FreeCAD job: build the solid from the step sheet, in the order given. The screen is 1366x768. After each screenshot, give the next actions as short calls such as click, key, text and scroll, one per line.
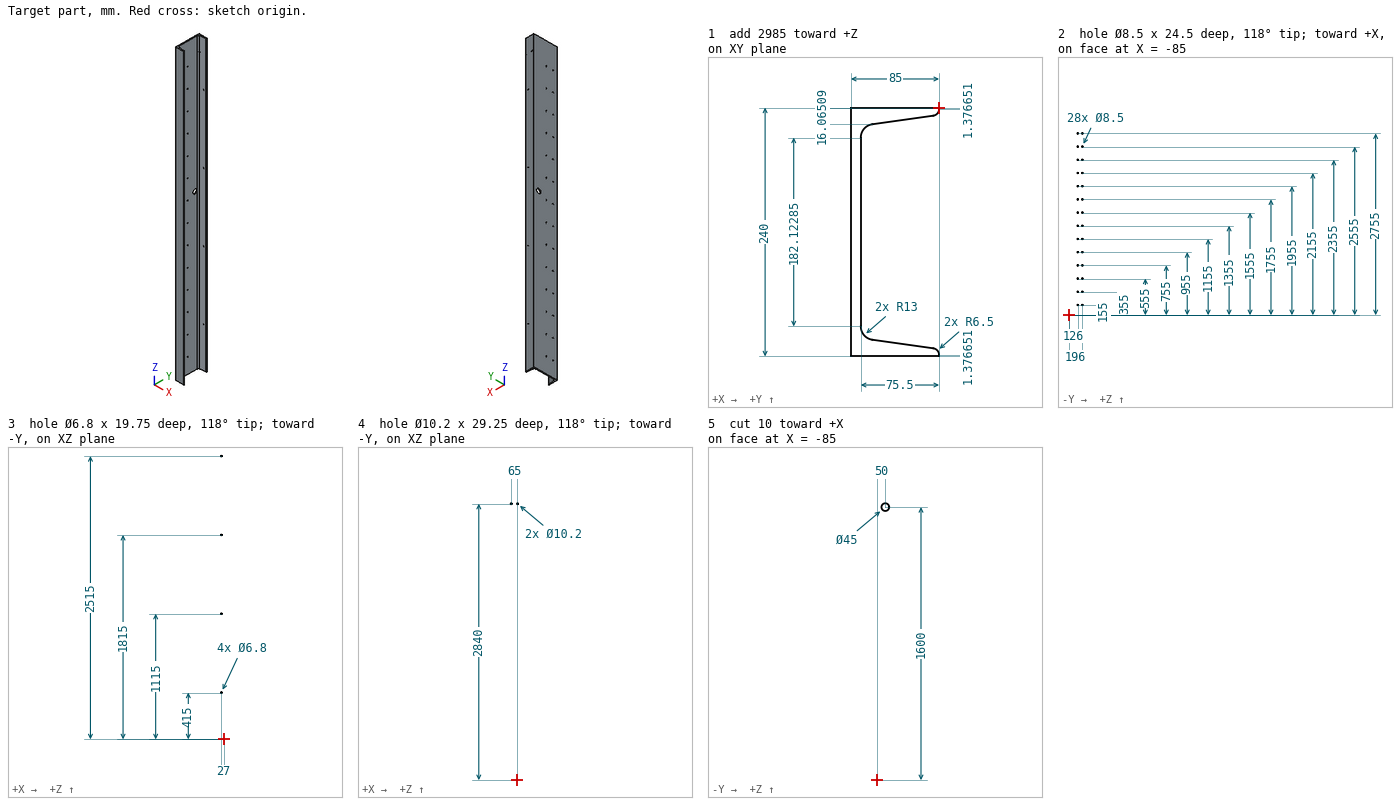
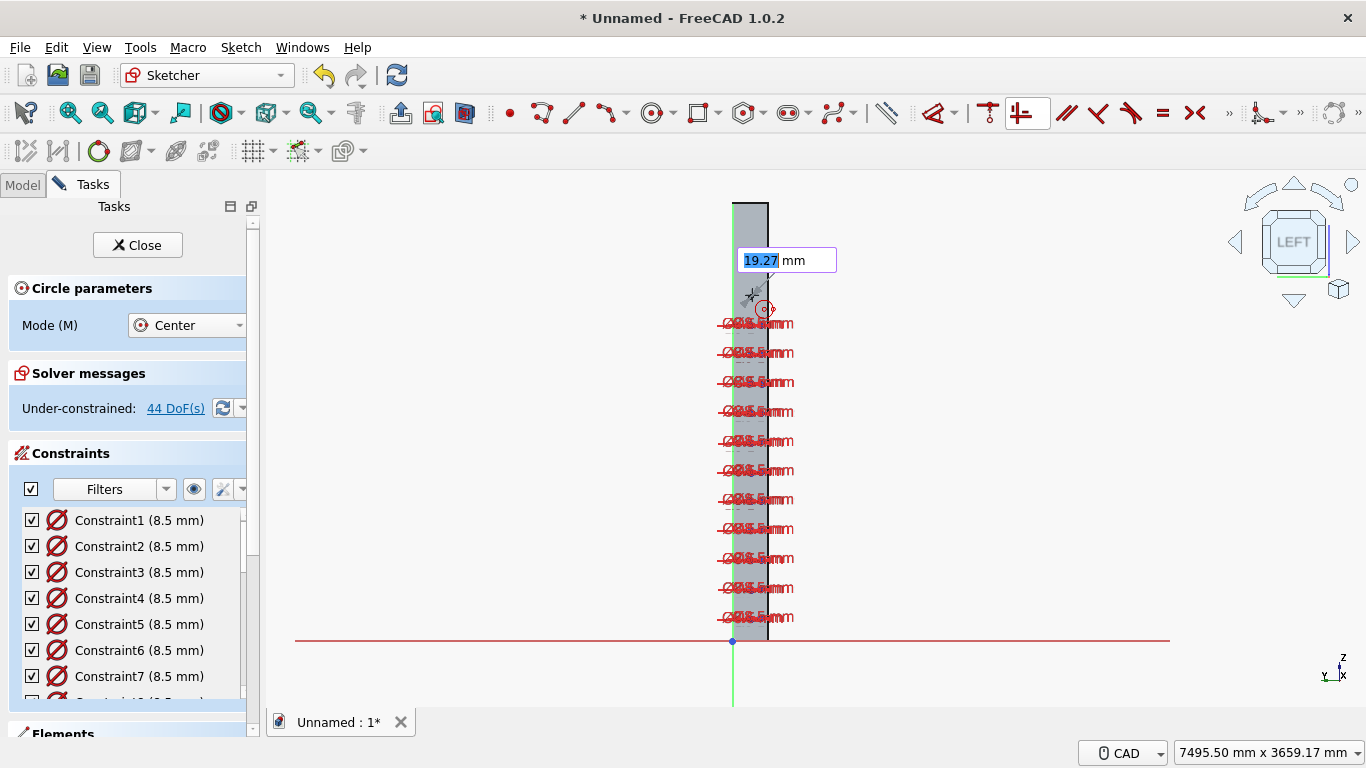
text(8.5)
key(Return)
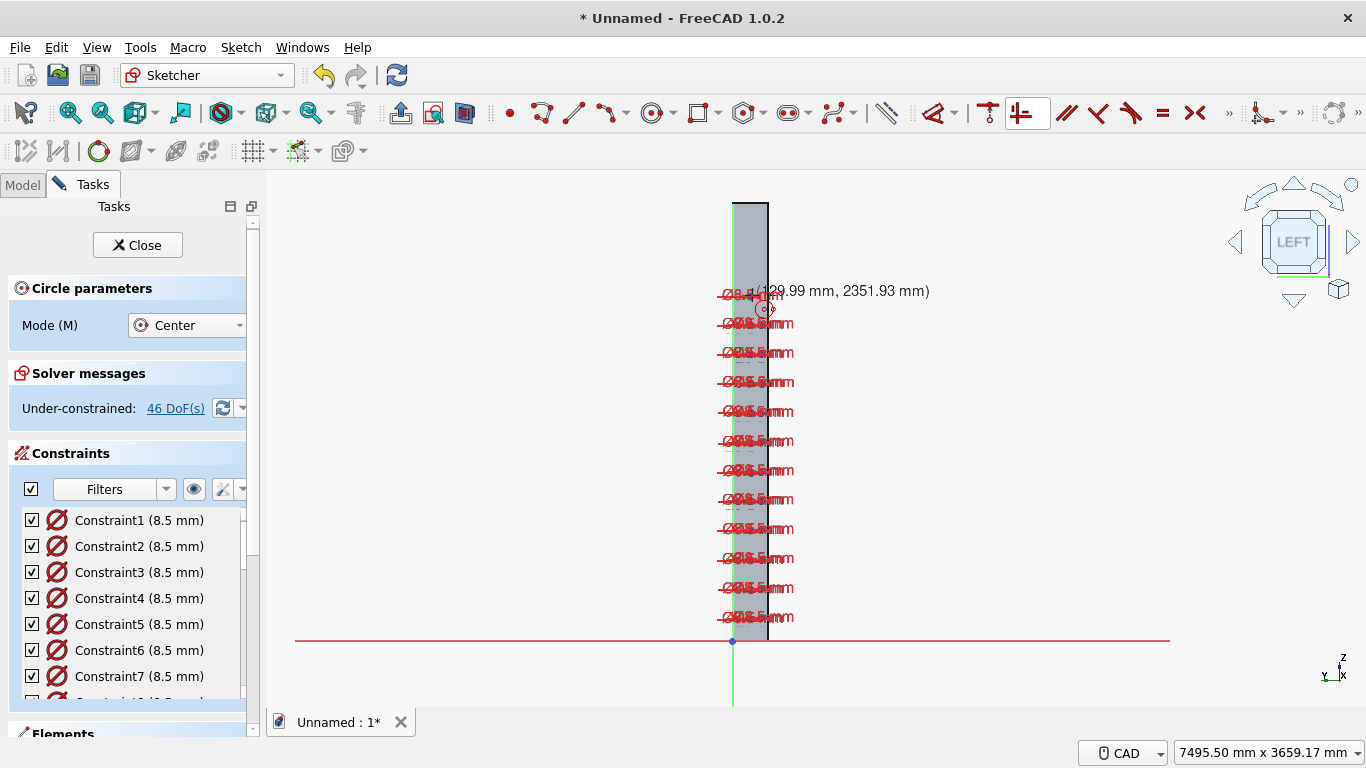
scroll(762, 296, up, 18)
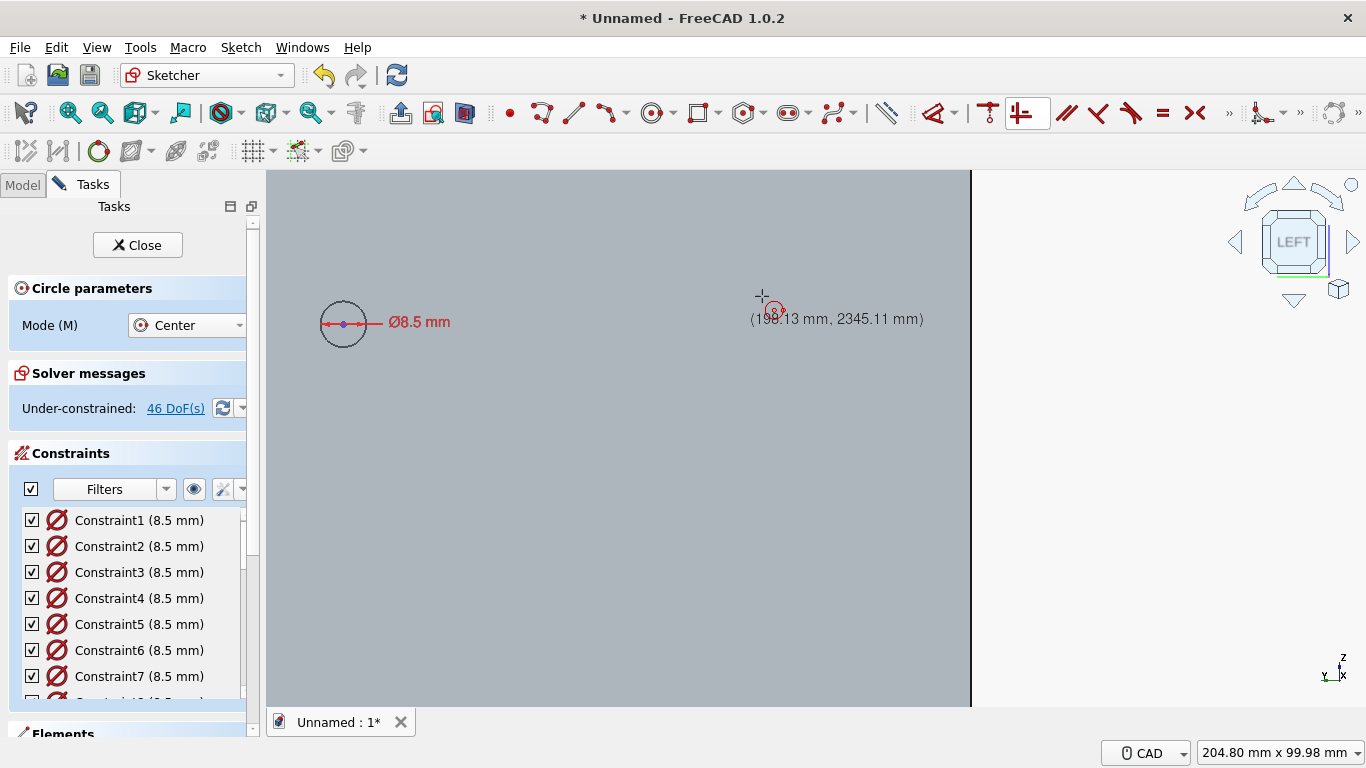
scroll(762, 296, down, 18)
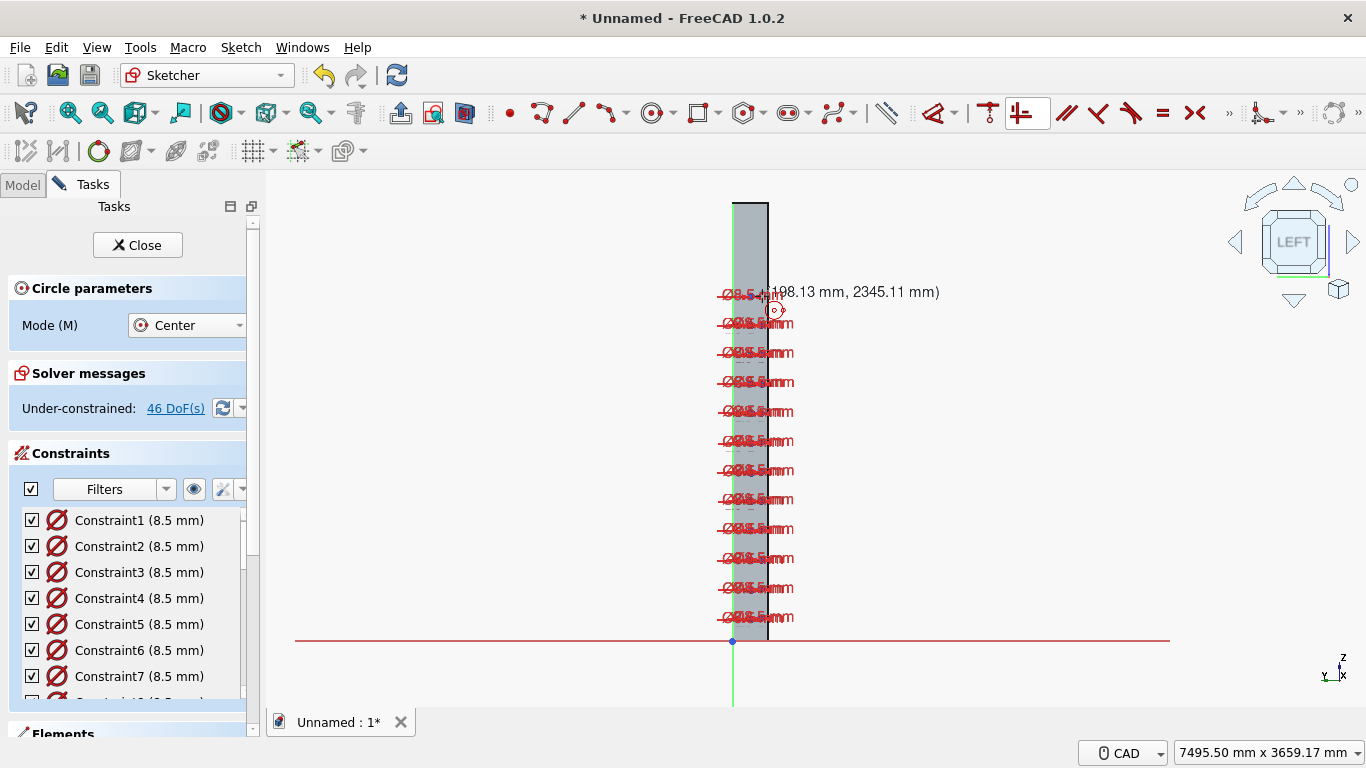
scroll(762, 296, up, 3)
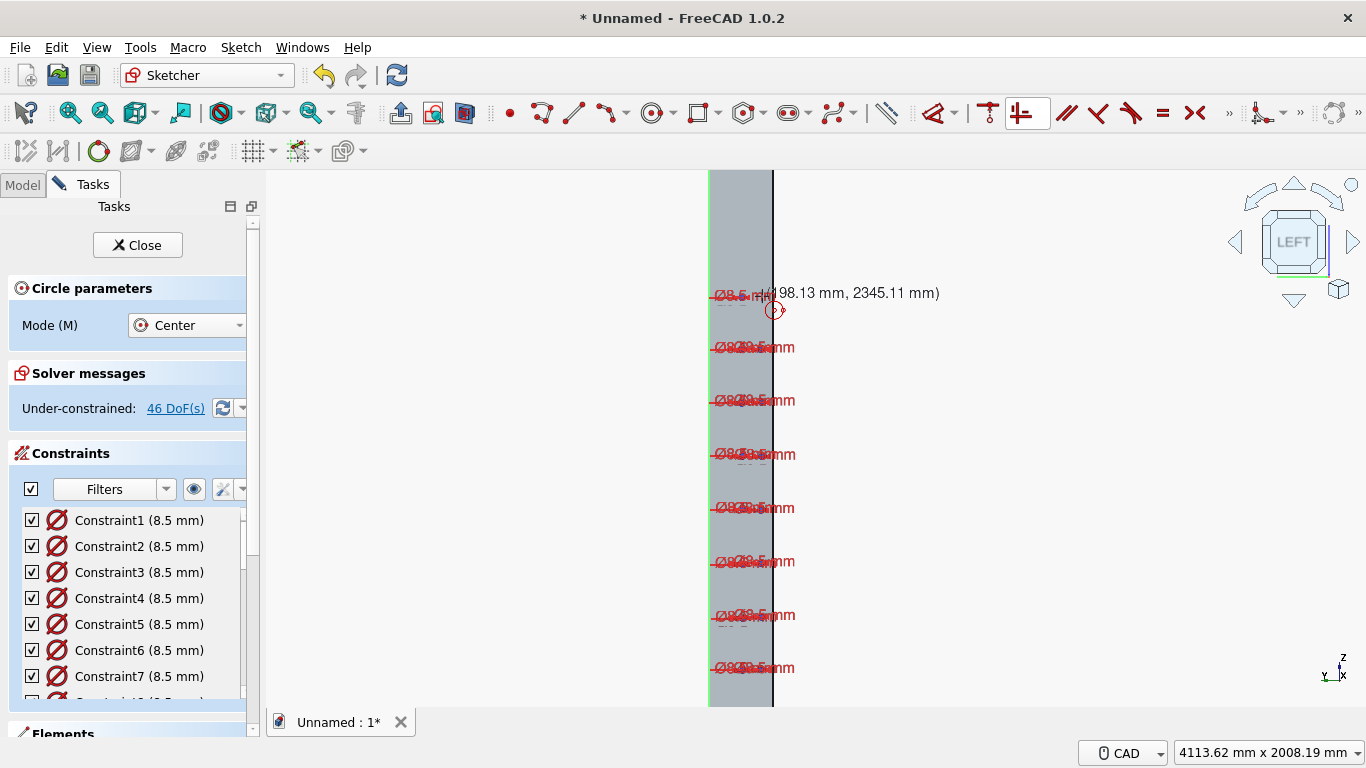
click(761, 295)
move(762, 294)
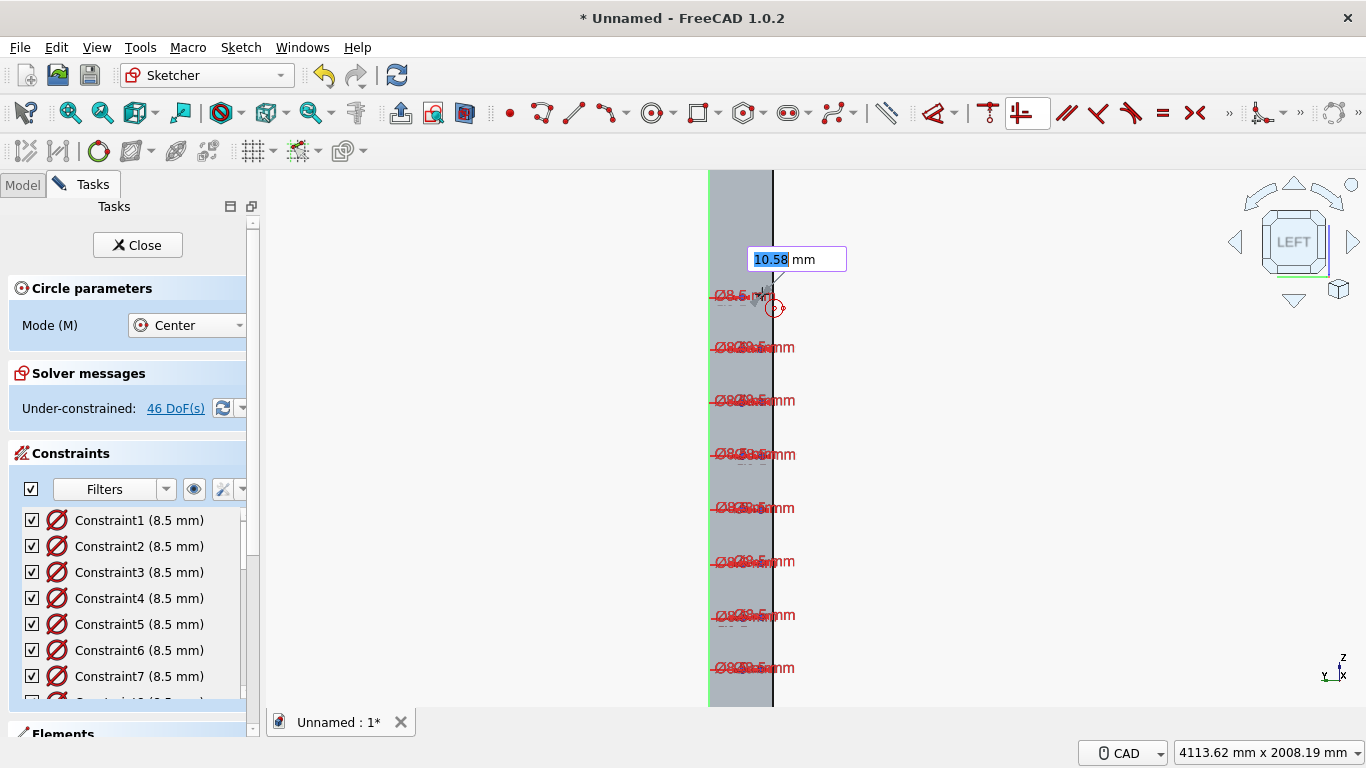
text(8.5)
key(Return)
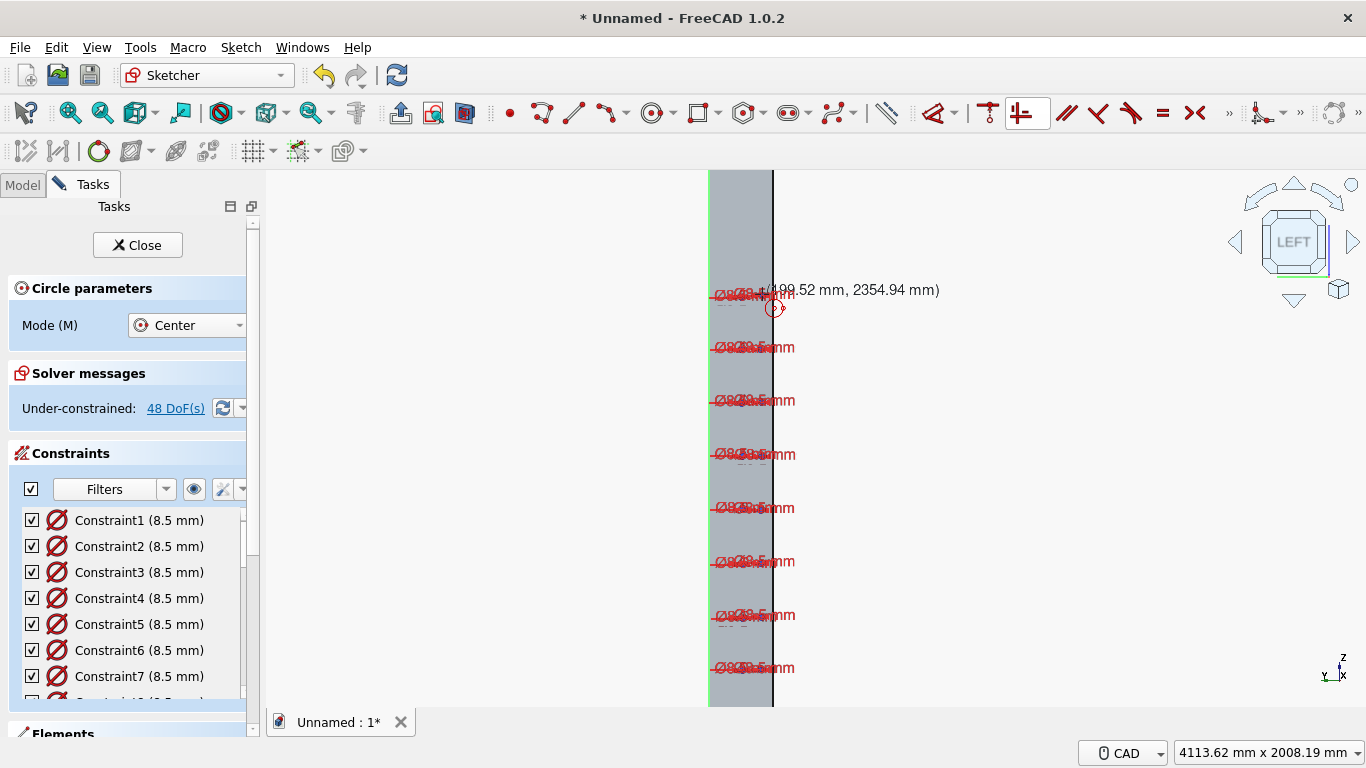
scroll(761, 242, up, 15)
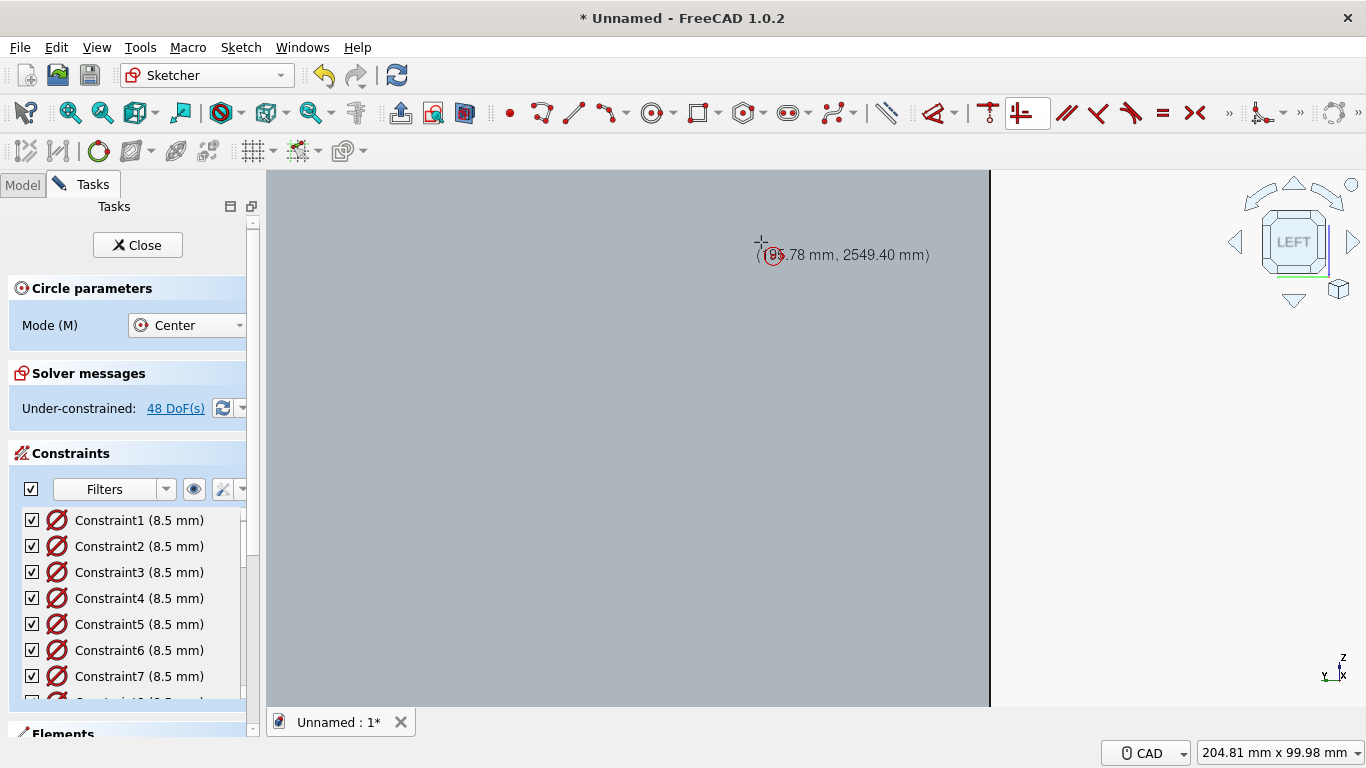
scroll(762, 267, down, 18)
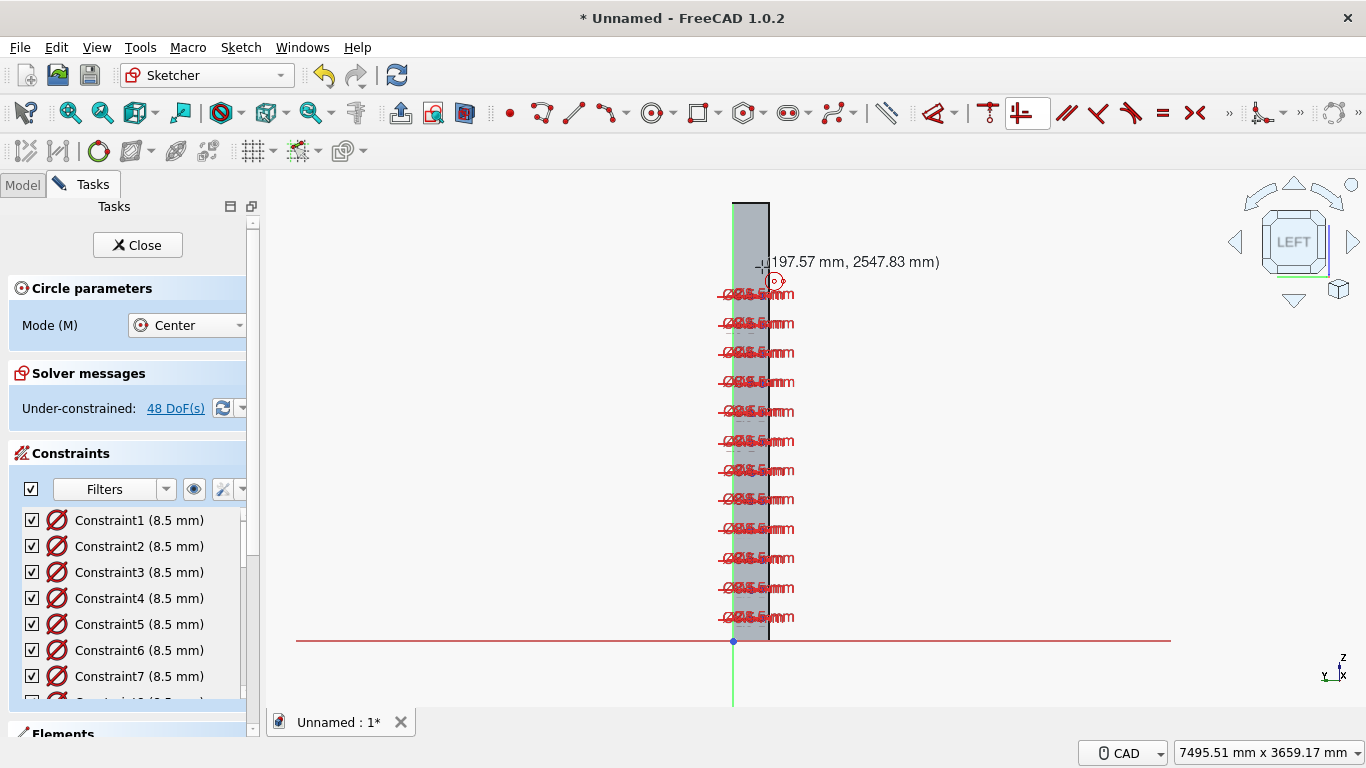
click(762, 266)
move(763, 266)